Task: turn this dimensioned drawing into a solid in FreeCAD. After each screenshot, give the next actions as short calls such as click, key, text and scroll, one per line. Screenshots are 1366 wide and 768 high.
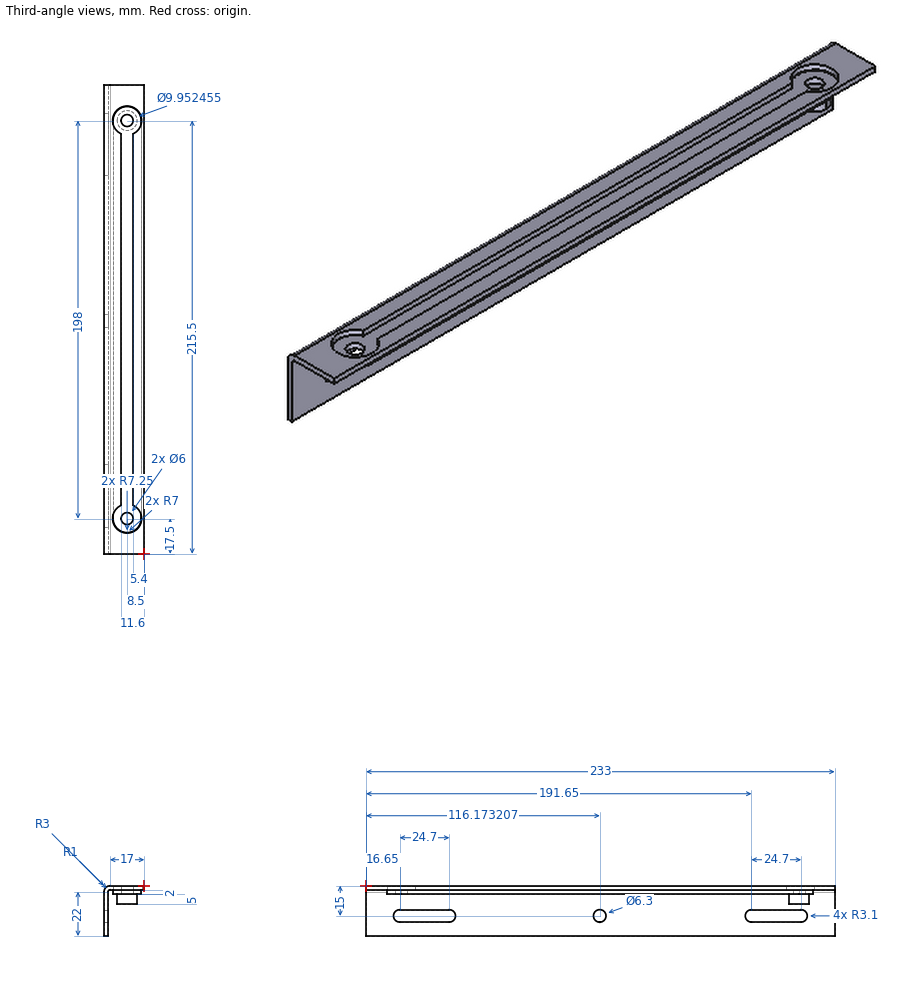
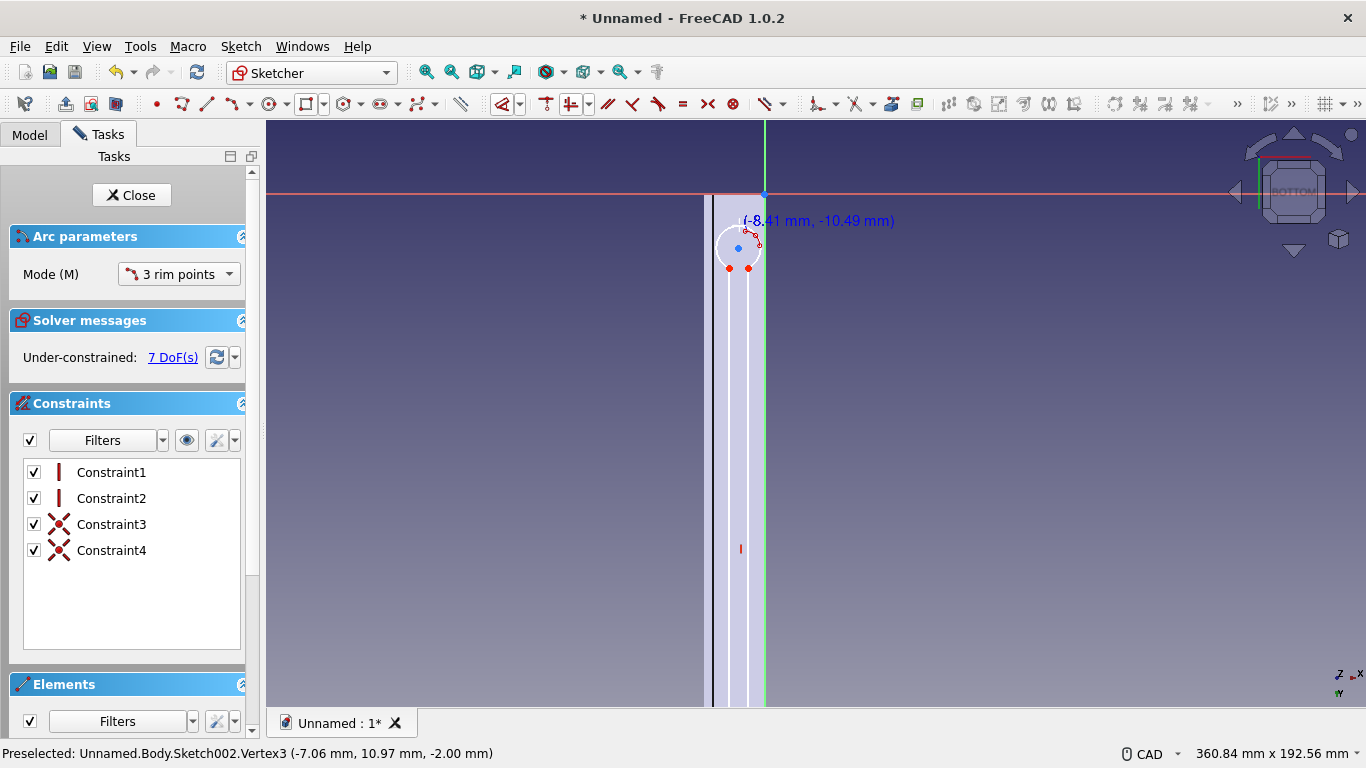
scroll(748, 267, down, 3)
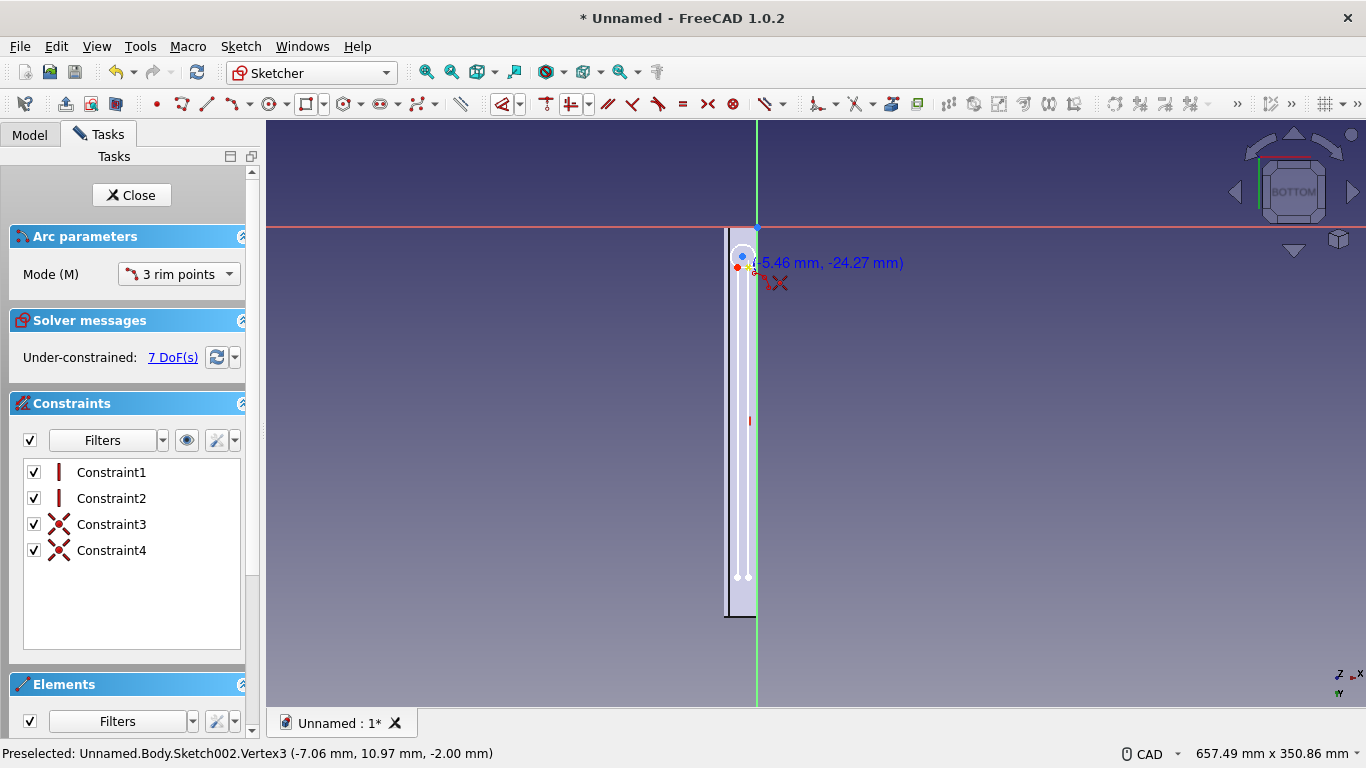
scroll(738, 577, up, 3)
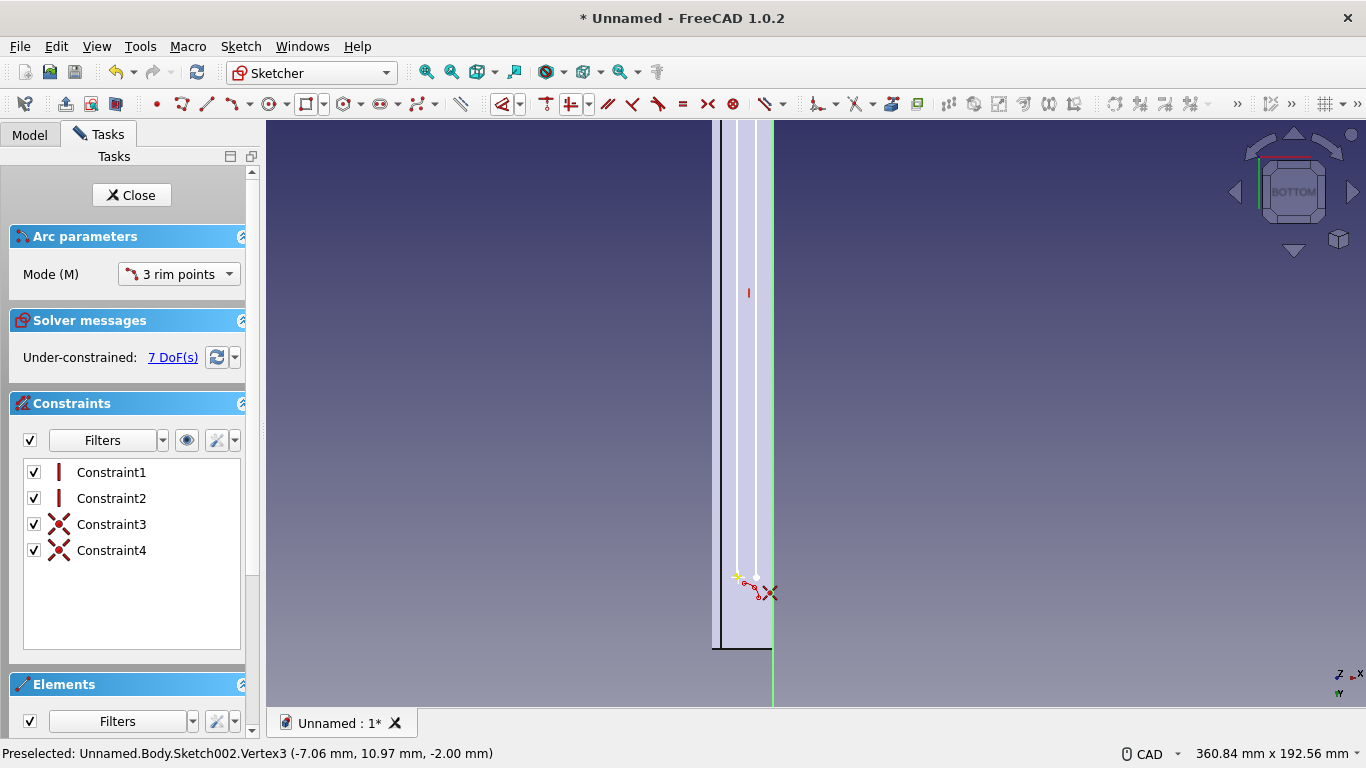
click(737, 577)
click(756, 577)
click(747, 618)
key(Escape)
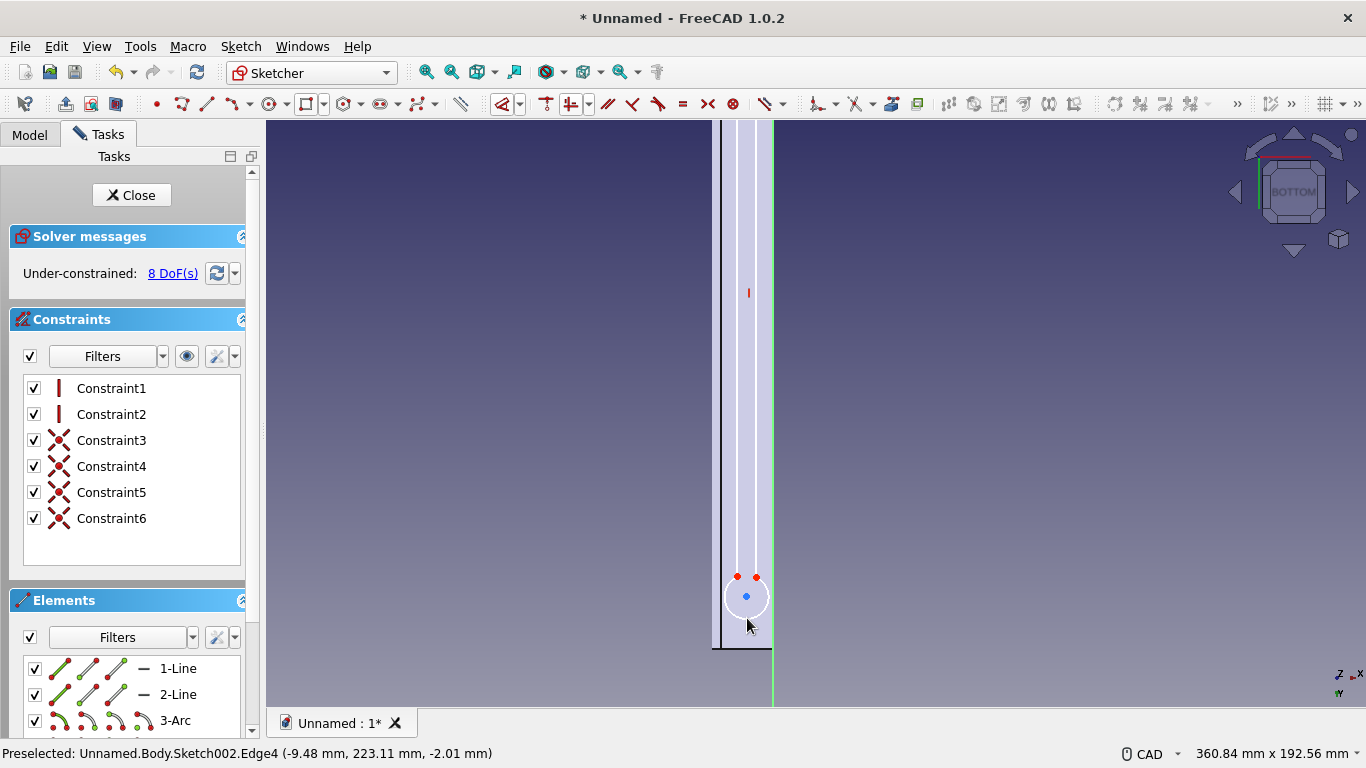
scroll(738, 578, down, 3)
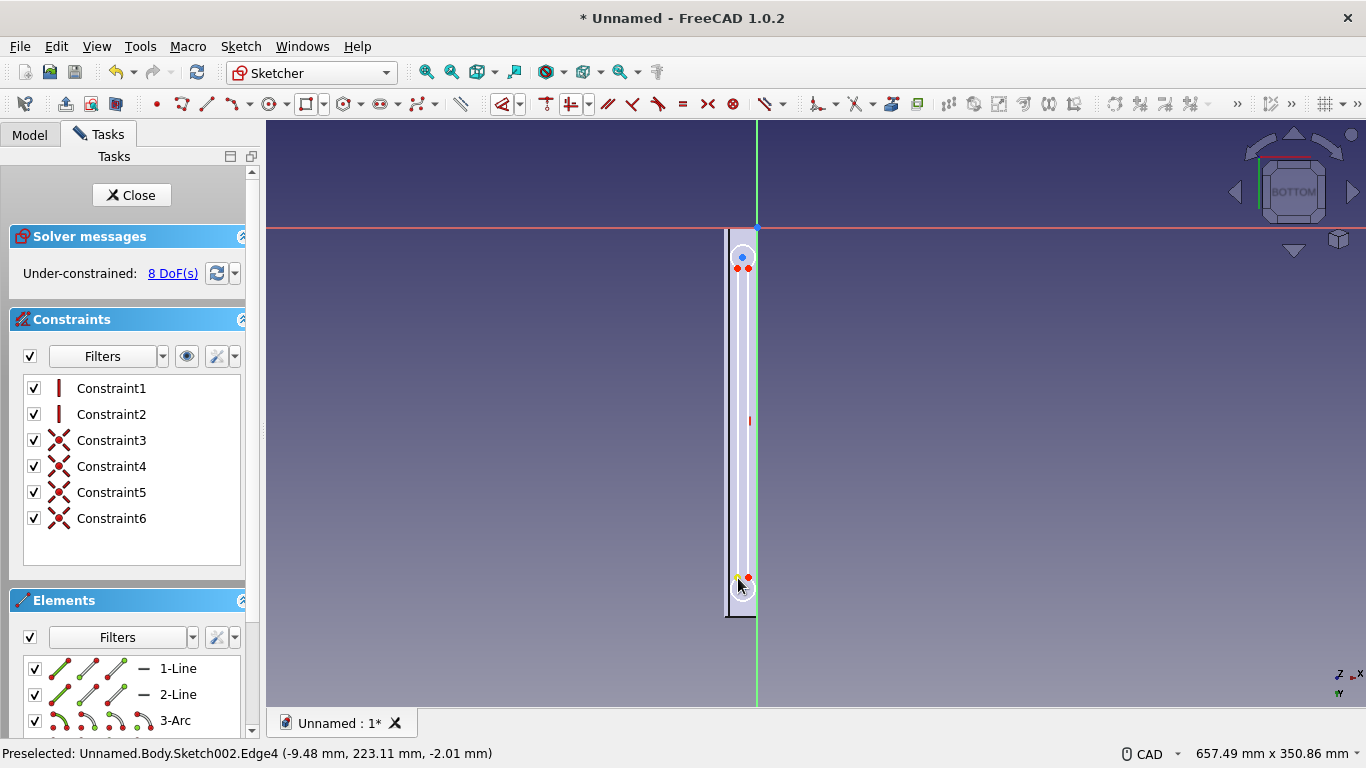
click(732, 251)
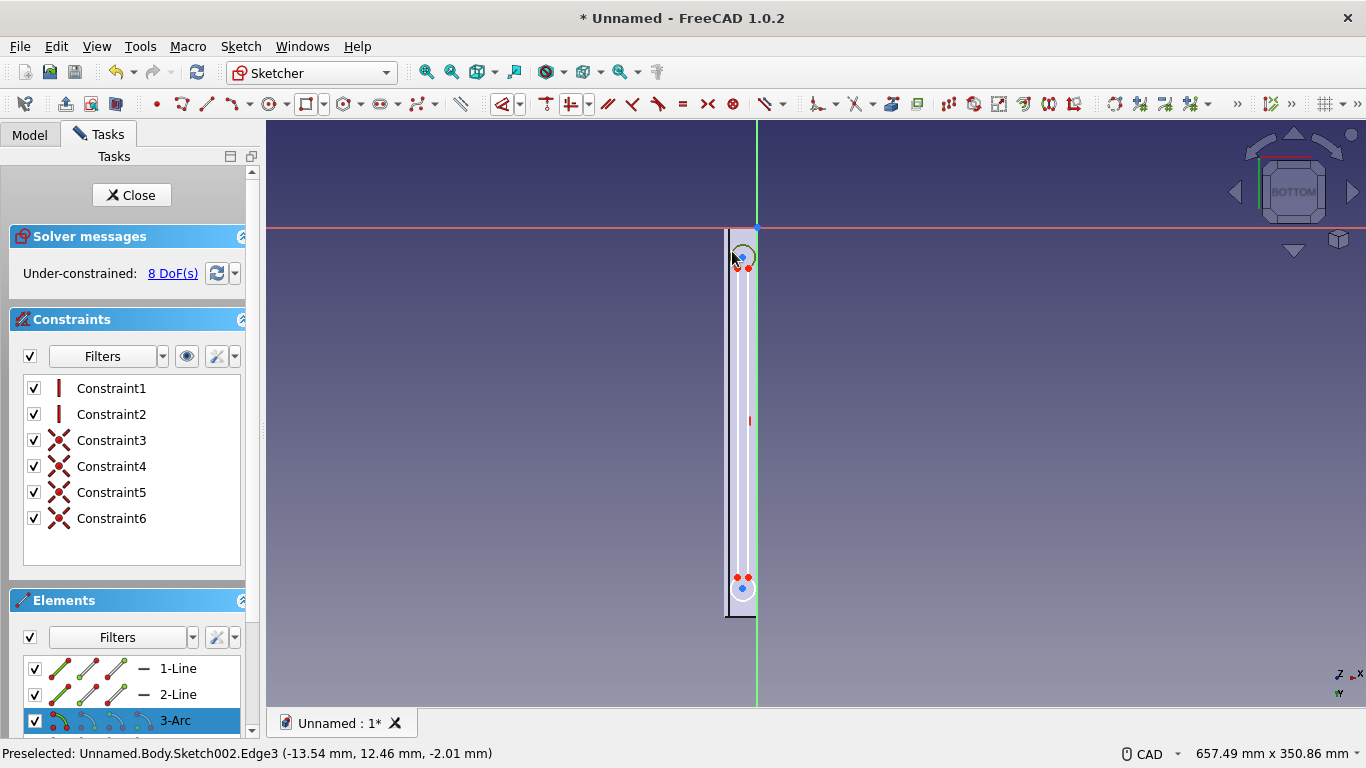
click(732, 594)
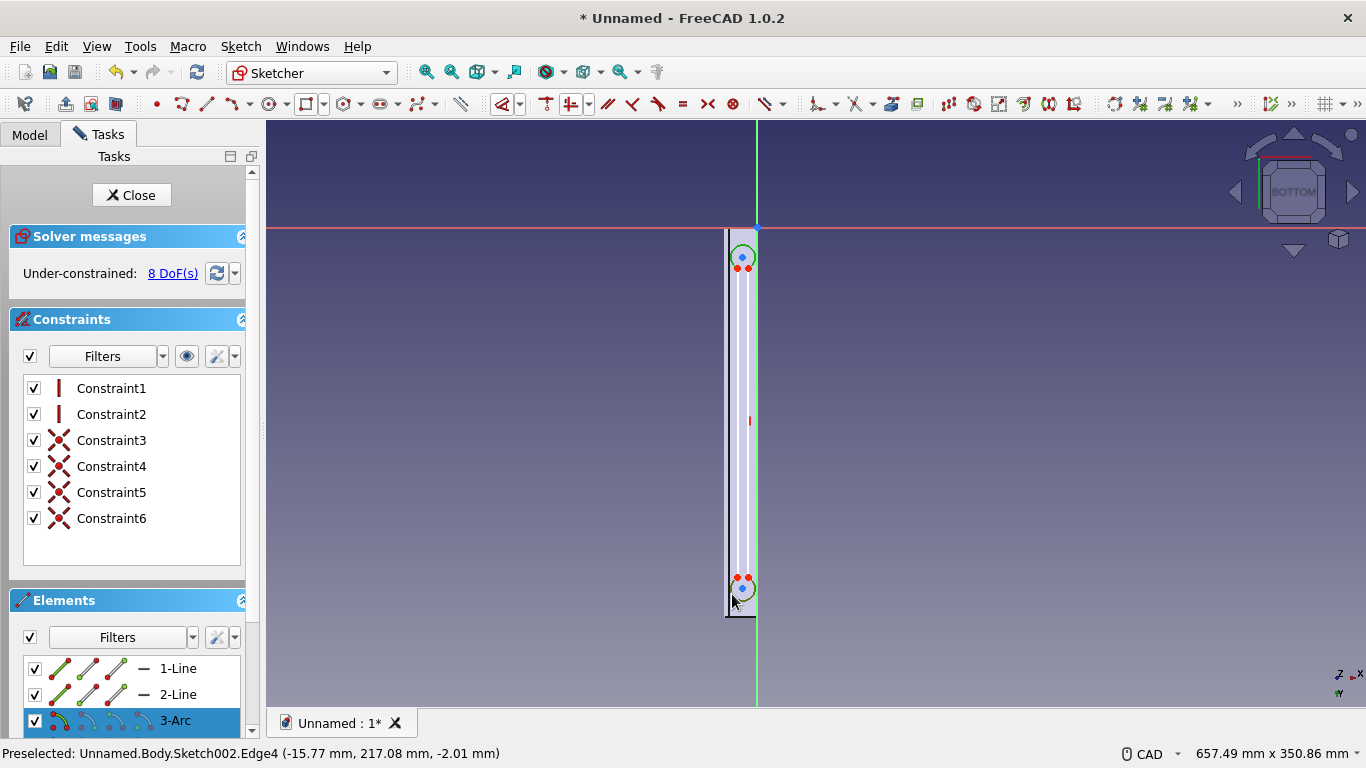
click(683, 104)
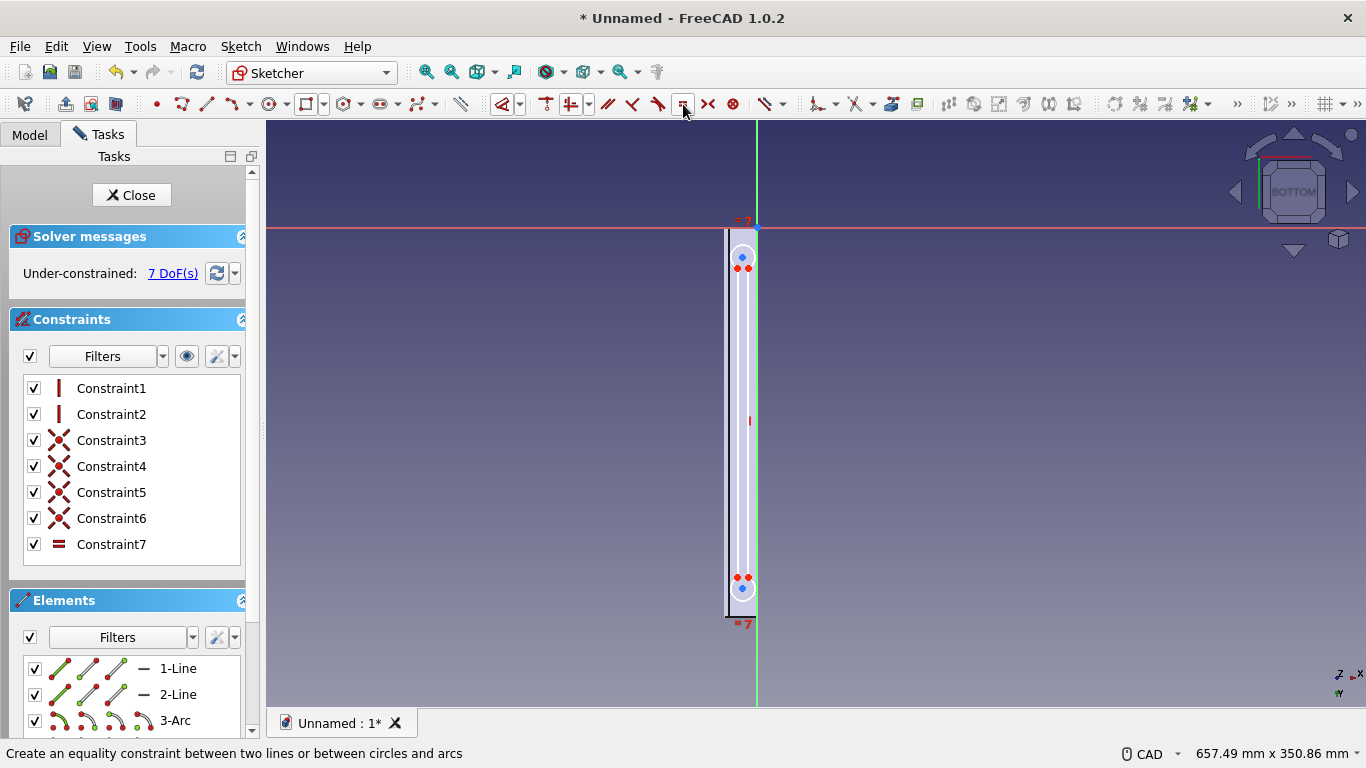
scroll(754, 251, up, 6)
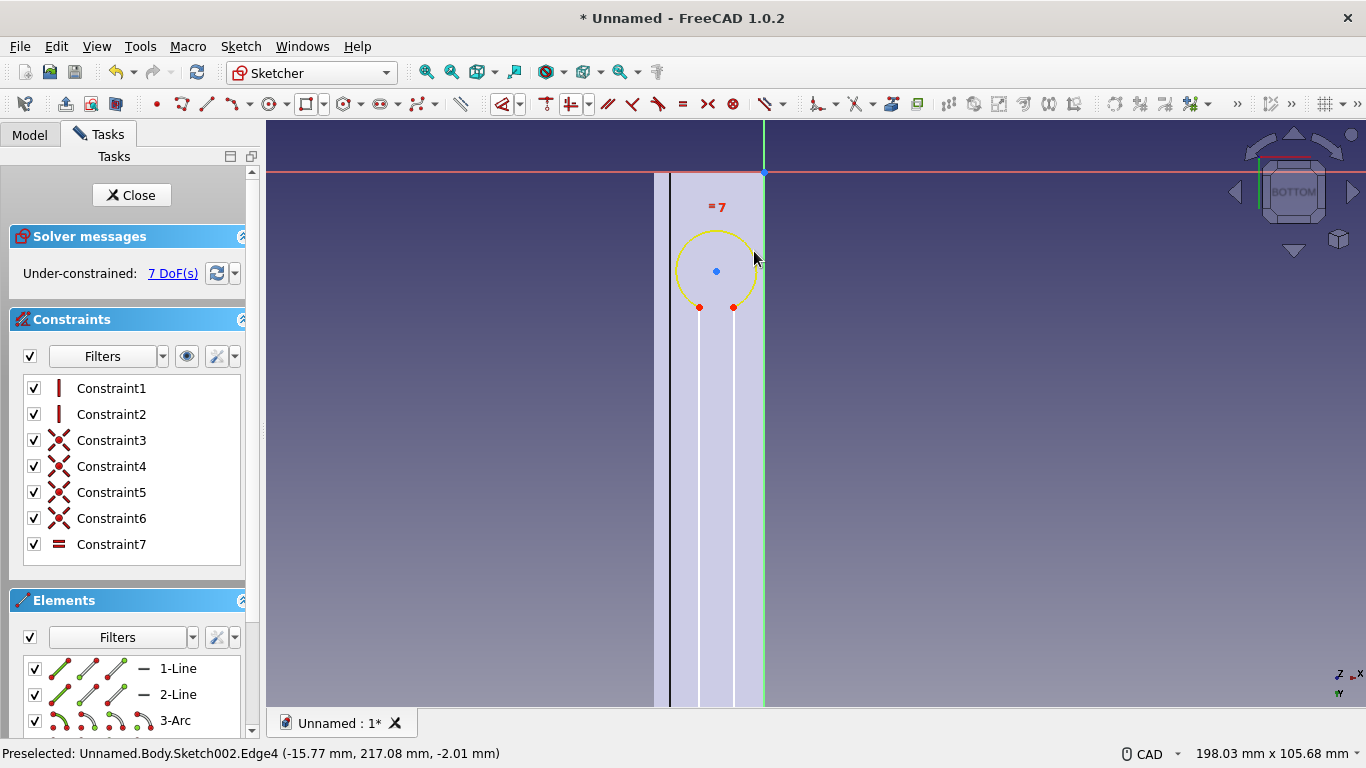
click(752, 252)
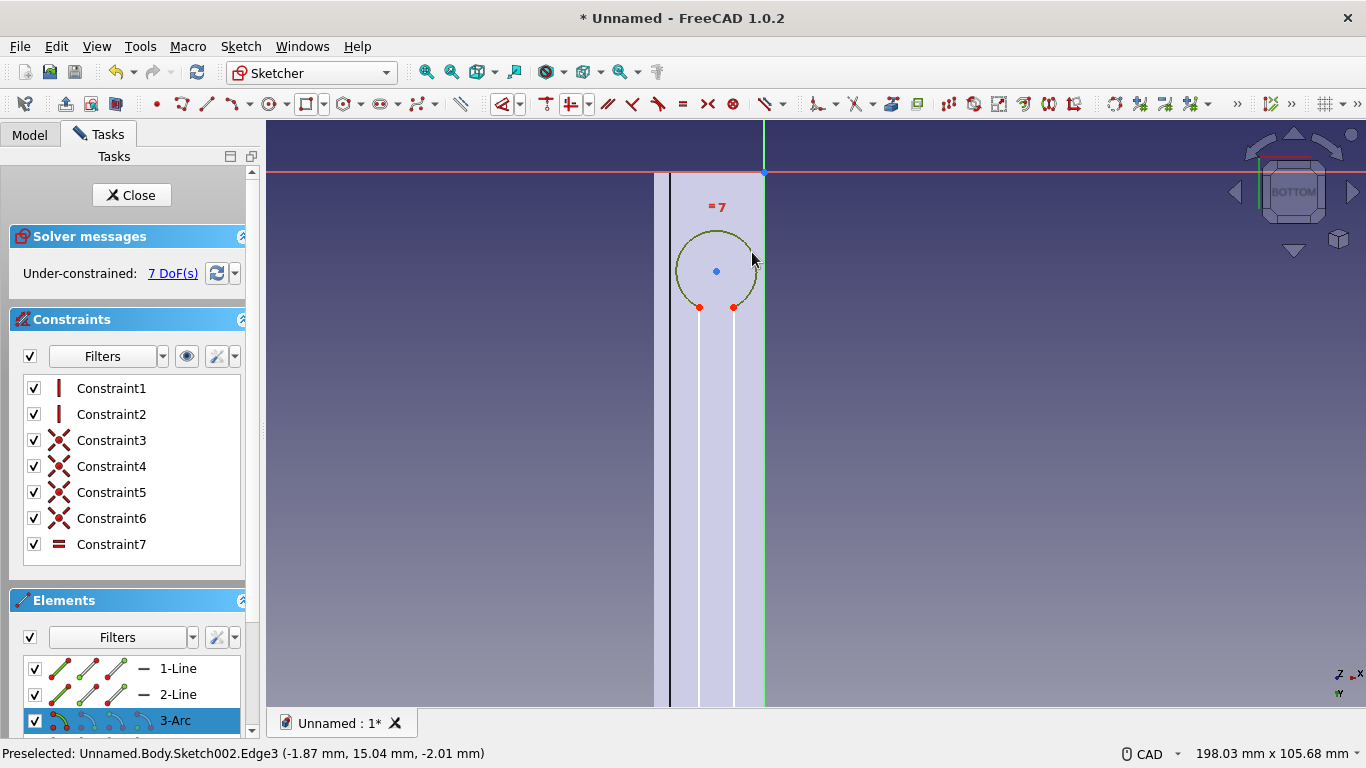
key(k)
key(r)